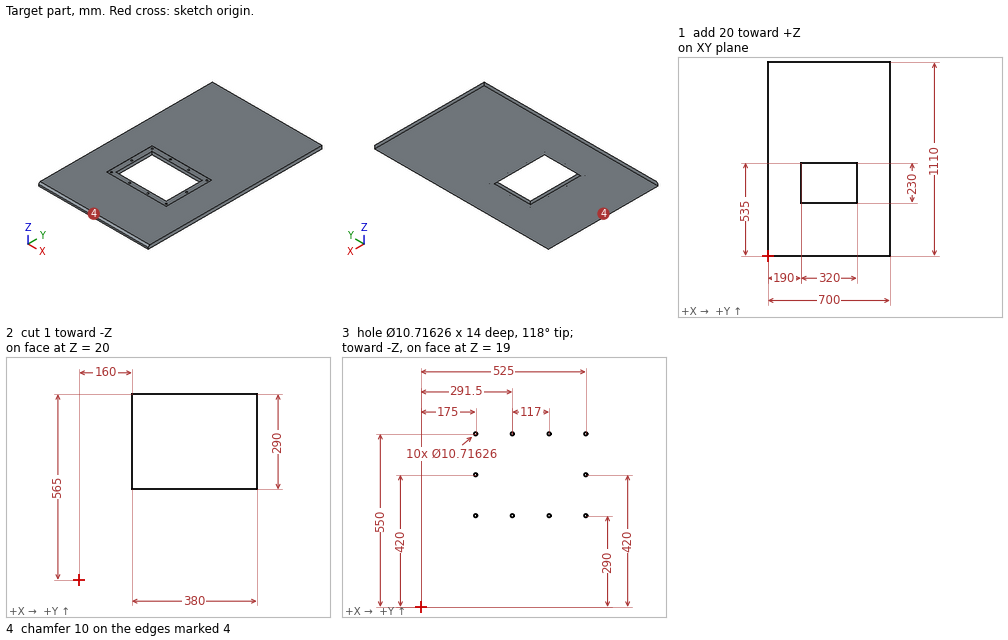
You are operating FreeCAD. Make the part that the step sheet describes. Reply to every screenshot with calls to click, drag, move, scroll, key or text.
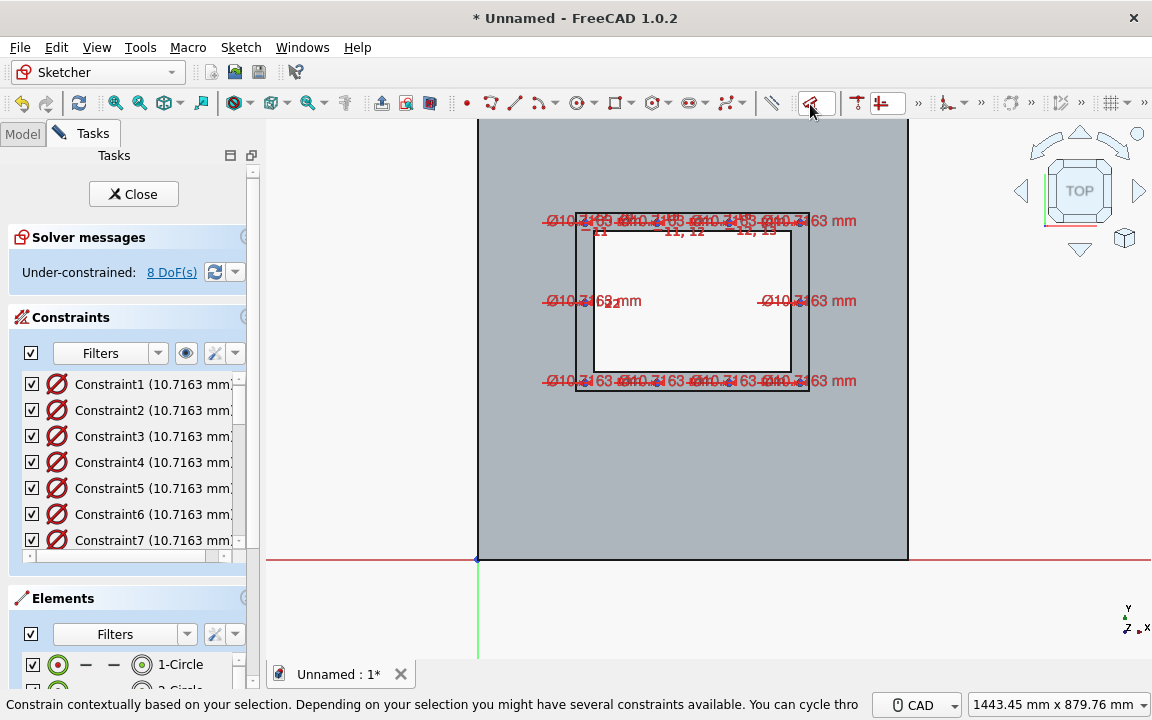
click(585, 223)
click(531, 594)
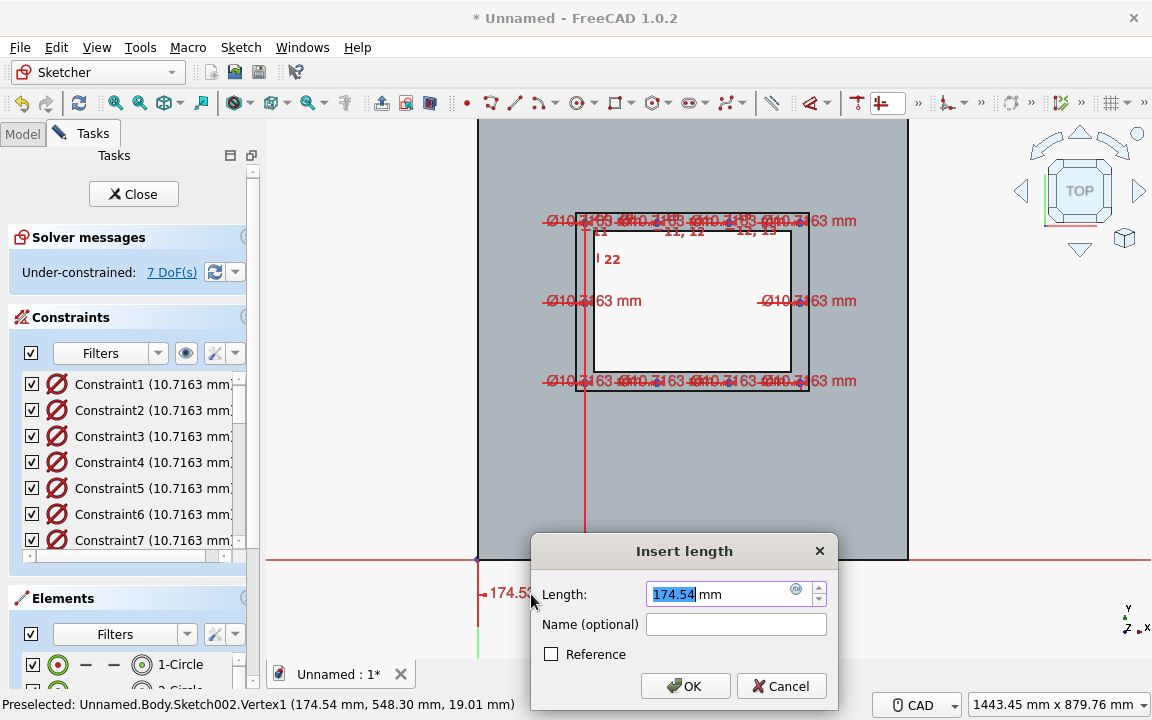
text(175)
key(Return)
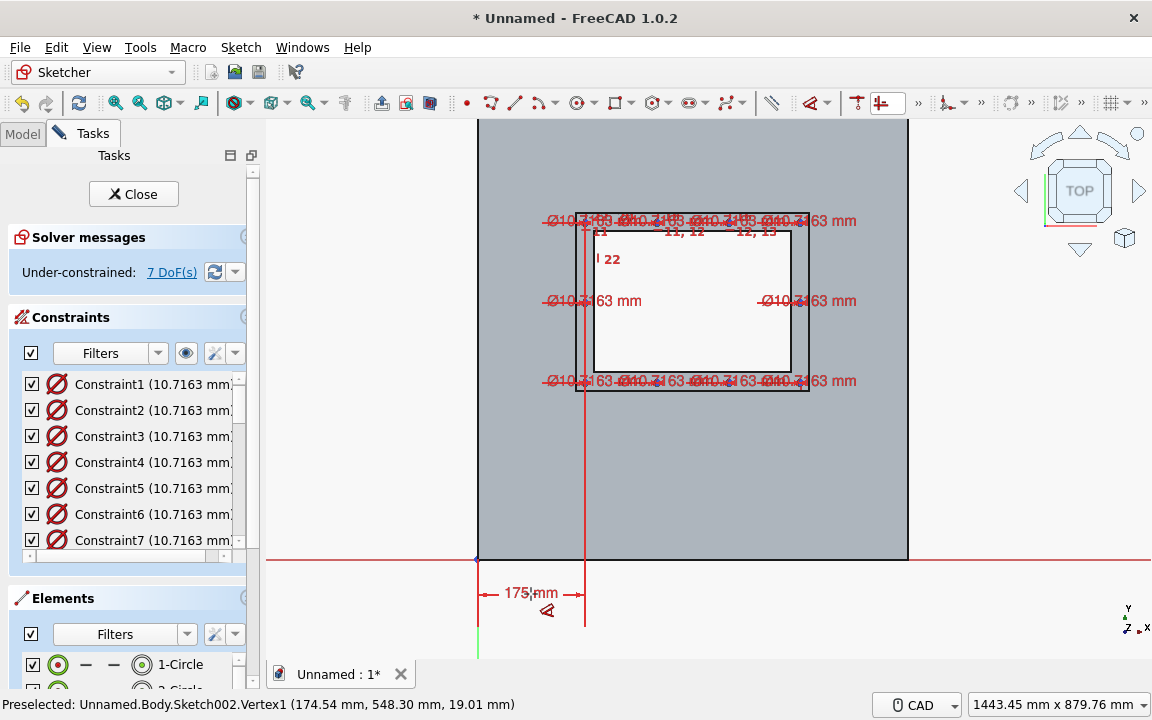
click(585, 223)
click(444, 391)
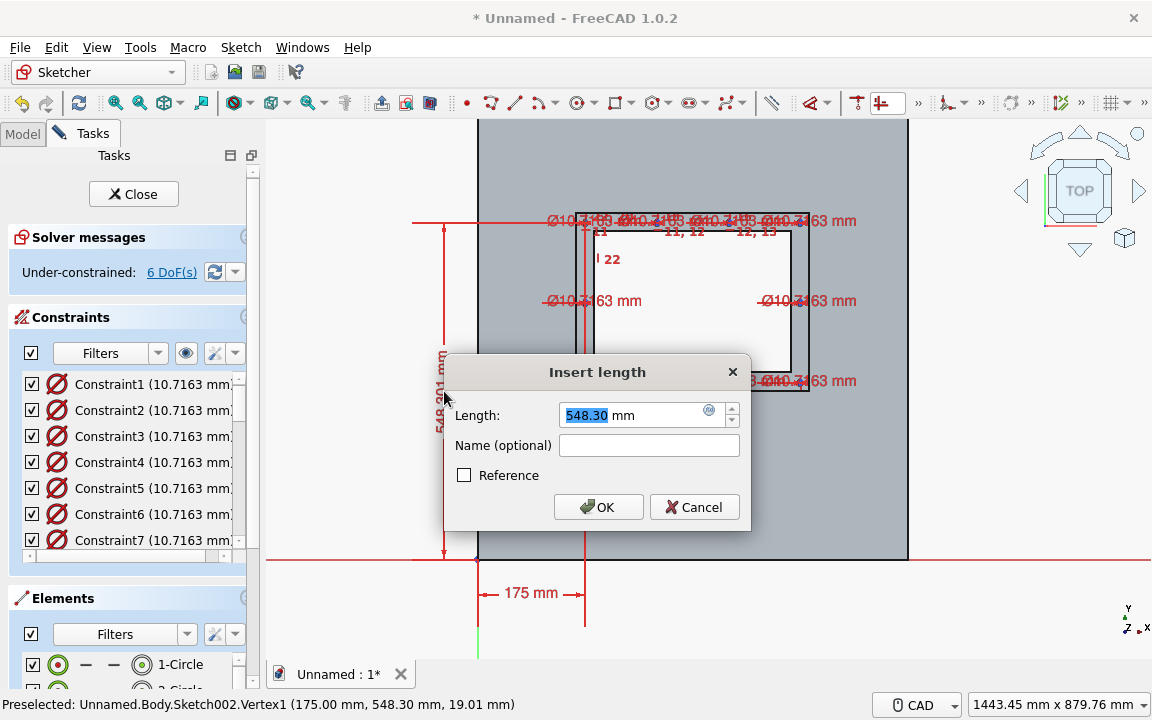
text(550)
key(Return)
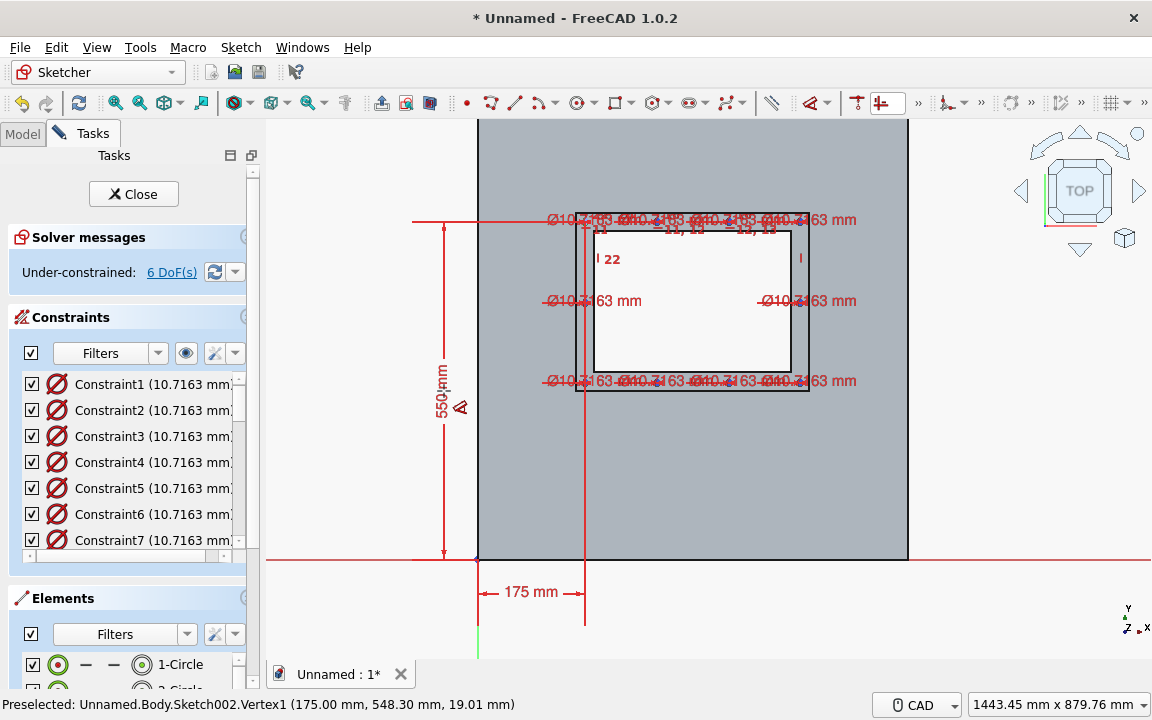
click(800, 222)
click(639, 594)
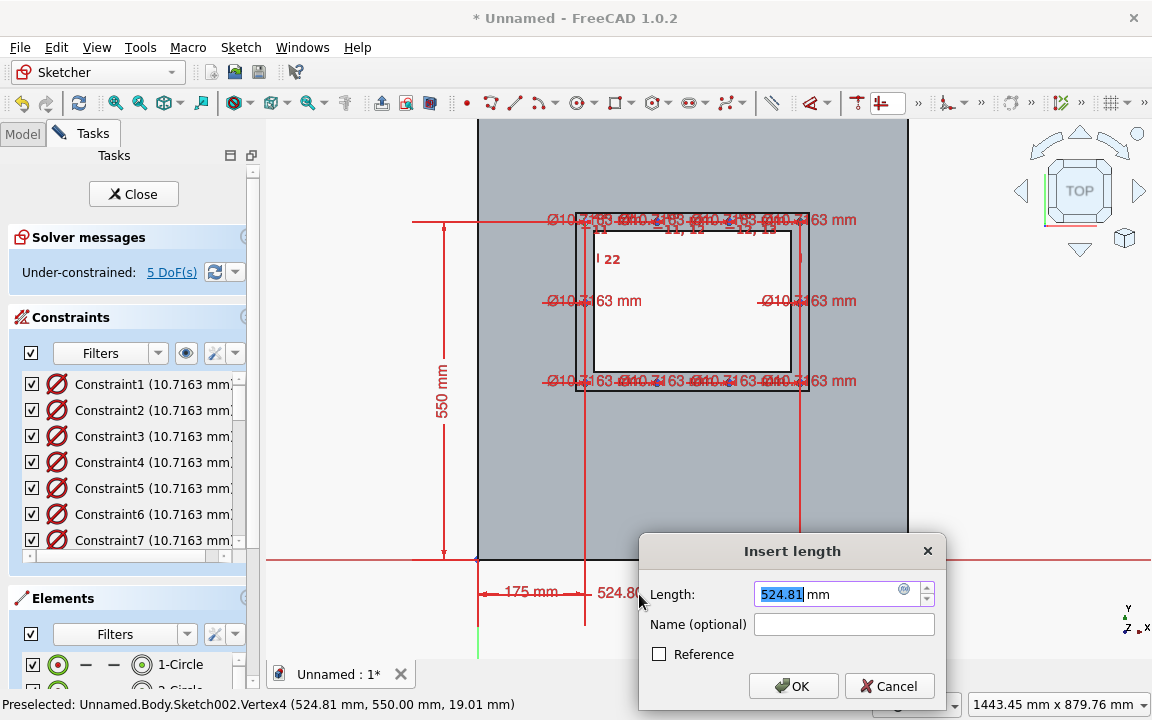
text(525)
key(Return)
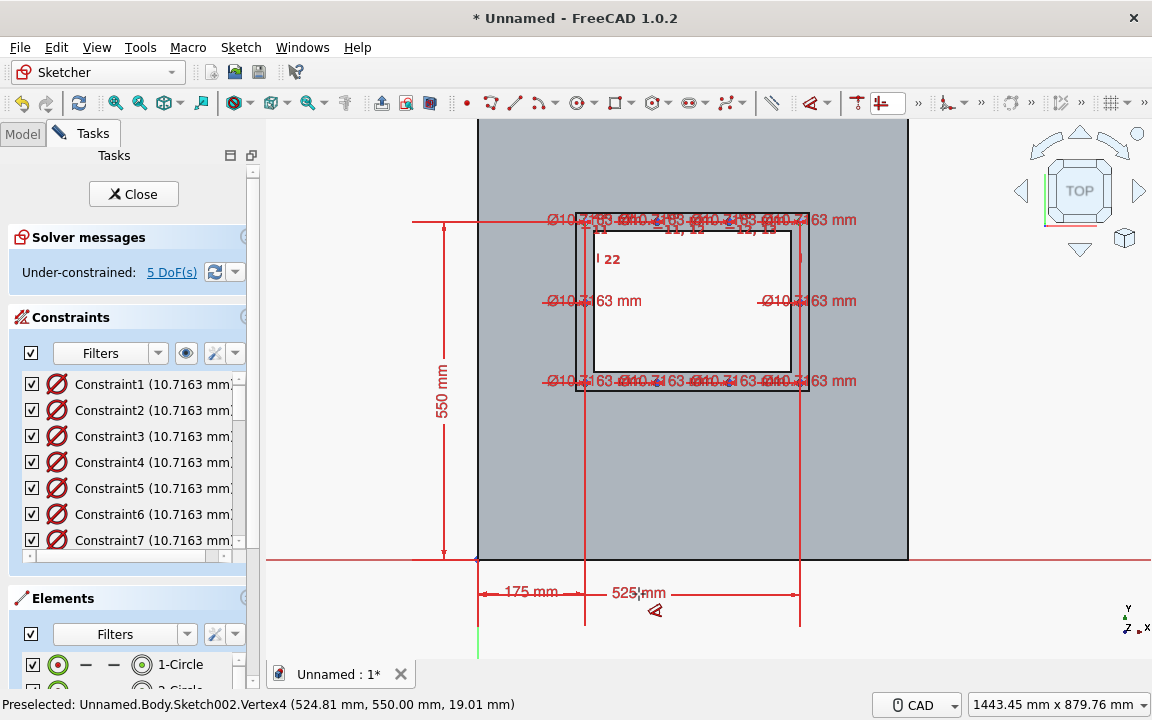
click(800, 303)
click(444, 431)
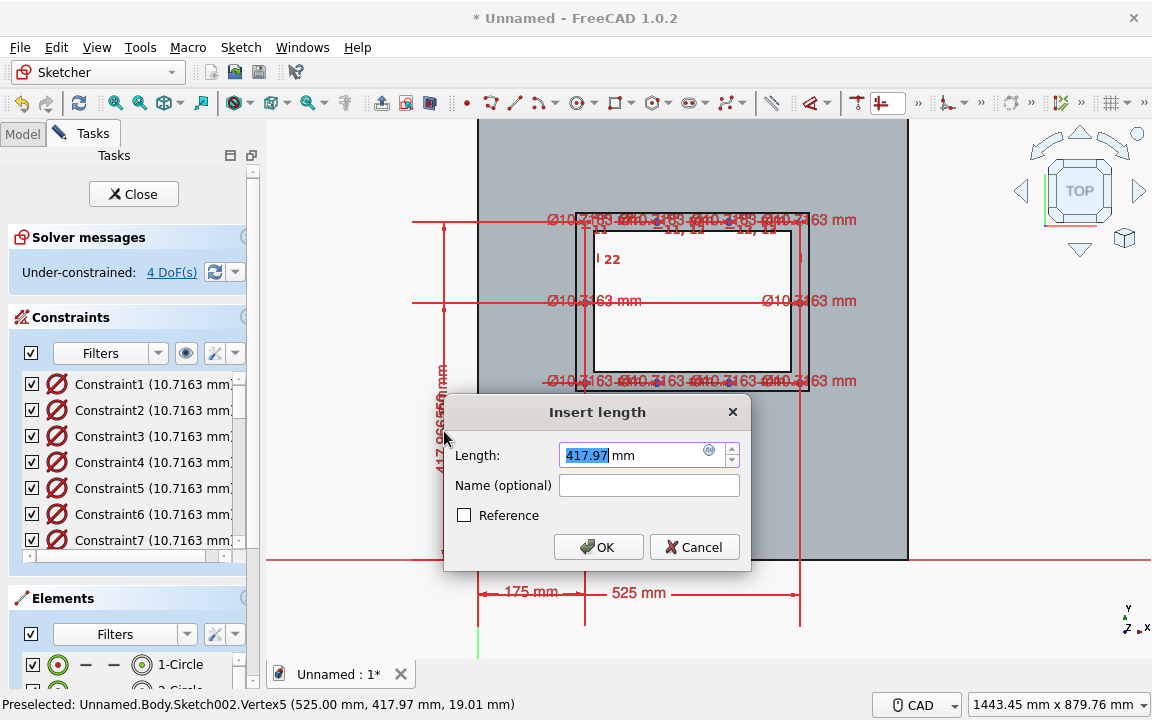
text(420)
key(Return)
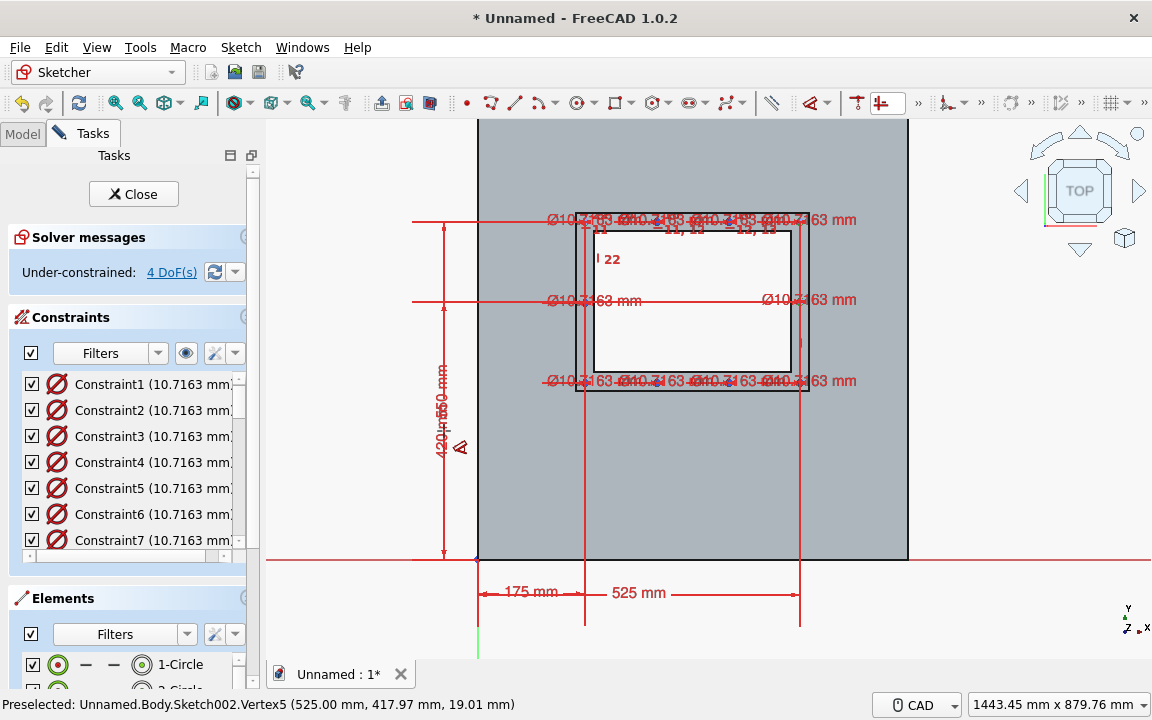
click(800, 383)
click(444, 471)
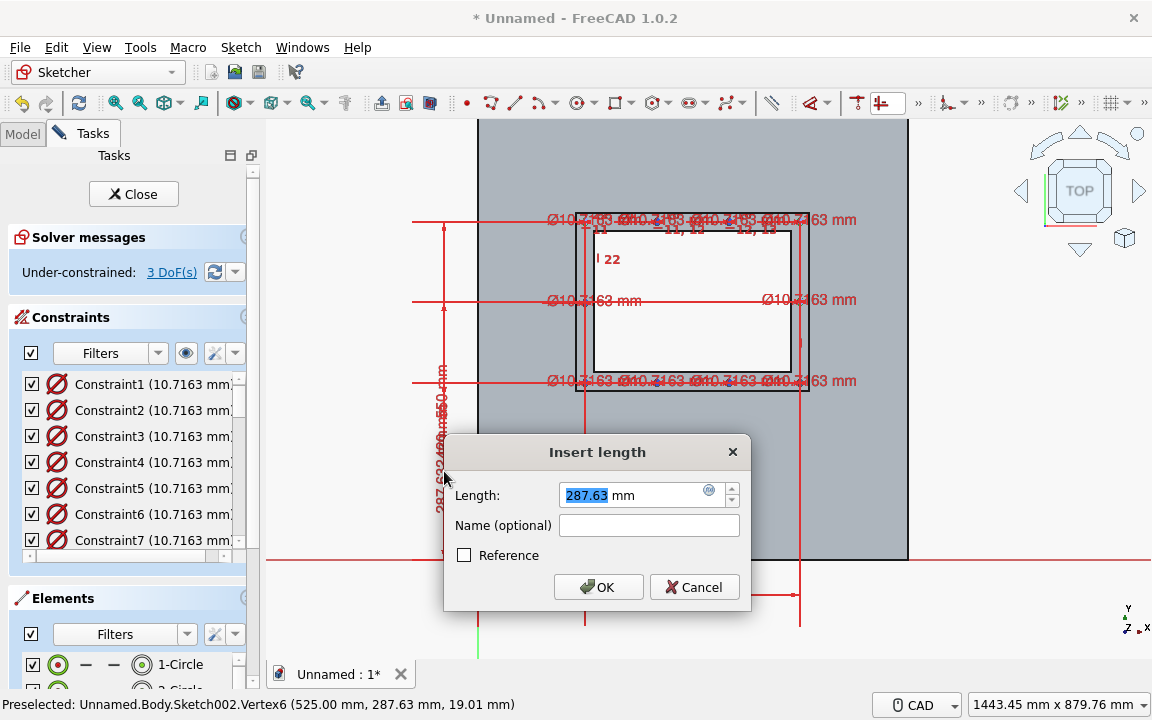
text(290)
key(Return)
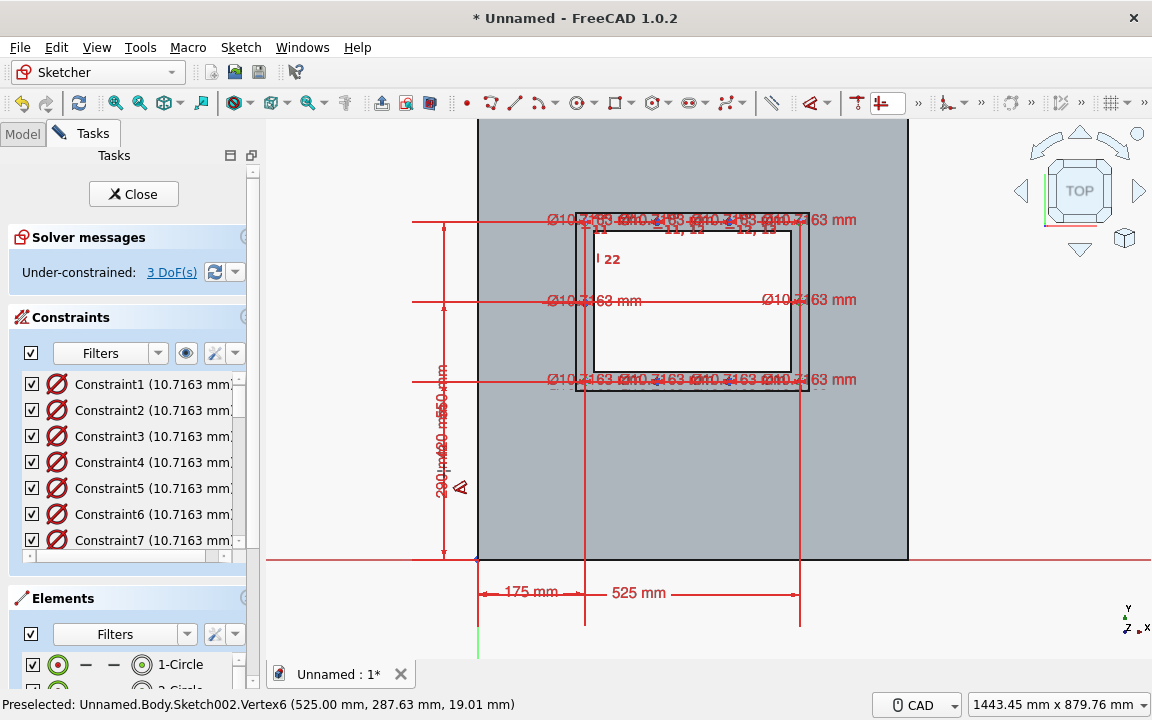
click(585, 303)
click(444, 341)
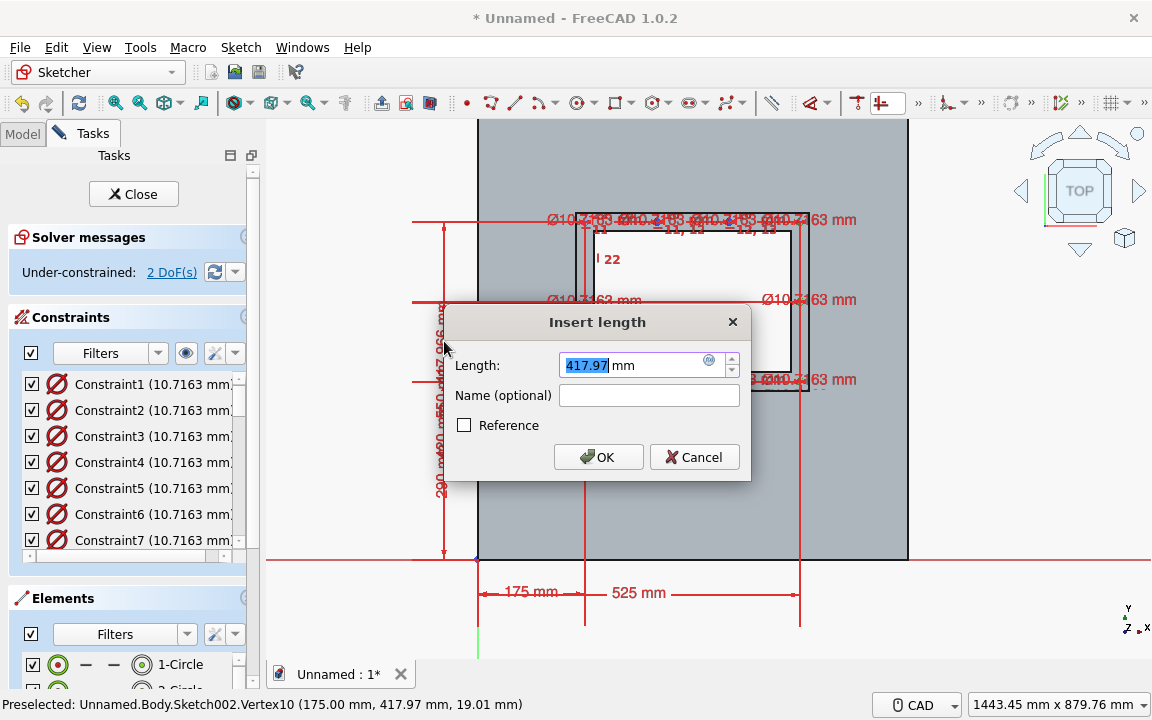
text(420)
key(Return)